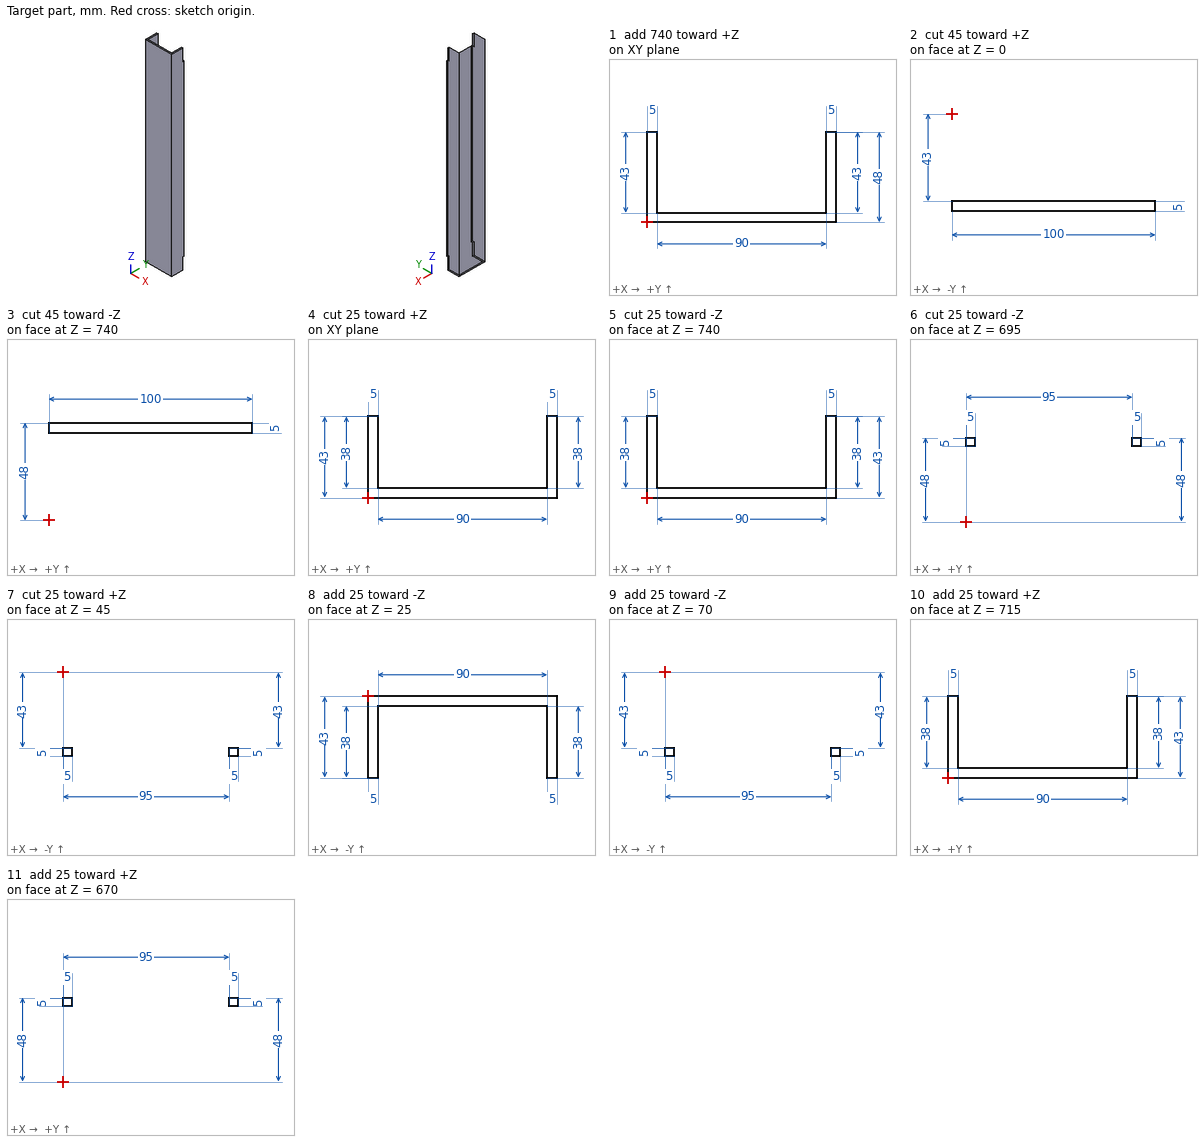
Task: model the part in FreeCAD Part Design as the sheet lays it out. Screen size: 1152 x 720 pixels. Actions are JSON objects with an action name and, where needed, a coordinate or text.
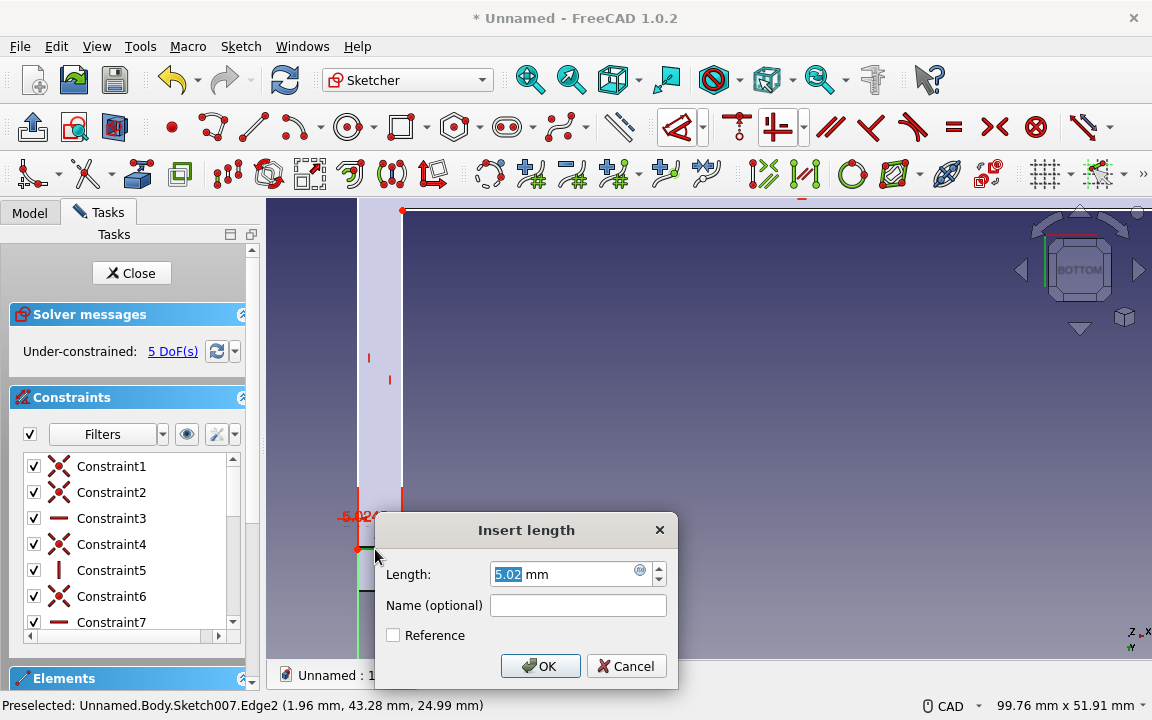
{"action": "type", "text": "5"}
{"action": "key", "text": "Return"}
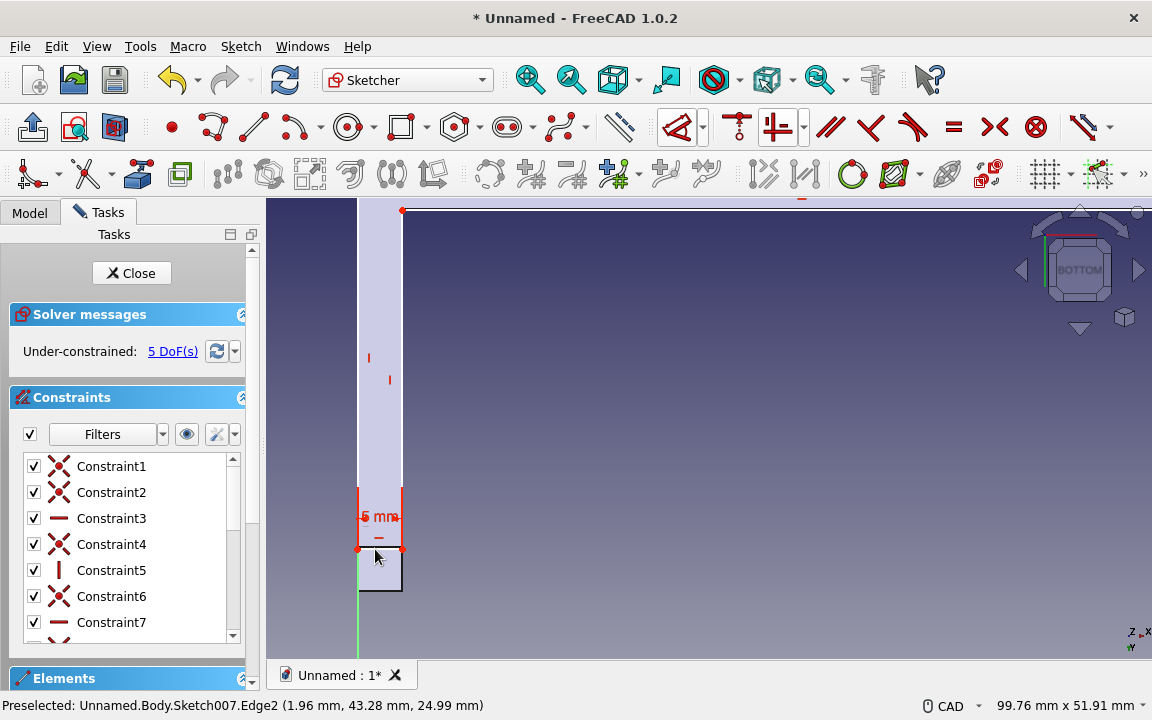
{"action": "scroll", "coordinate": [444, 517], "scroll_direction": "down", "scroll_amount": 3}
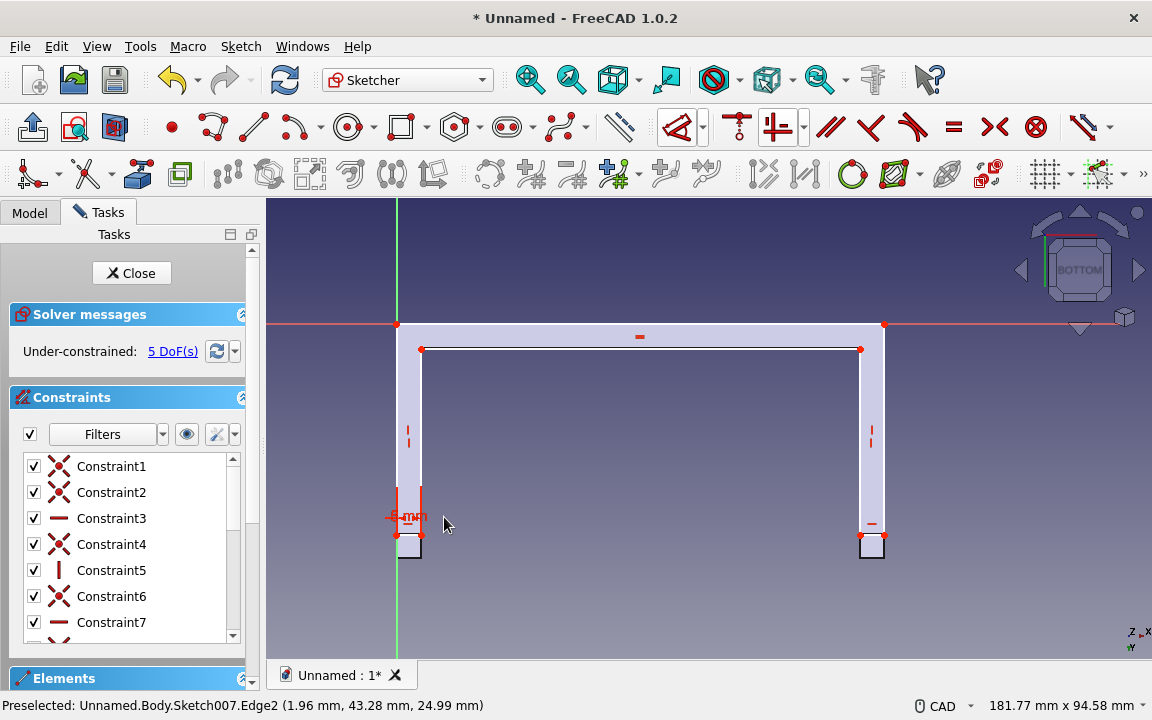
{"action": "scroll", "coordinate": [867, 535], "scroll_direction": "up", "scroll_amount": 4}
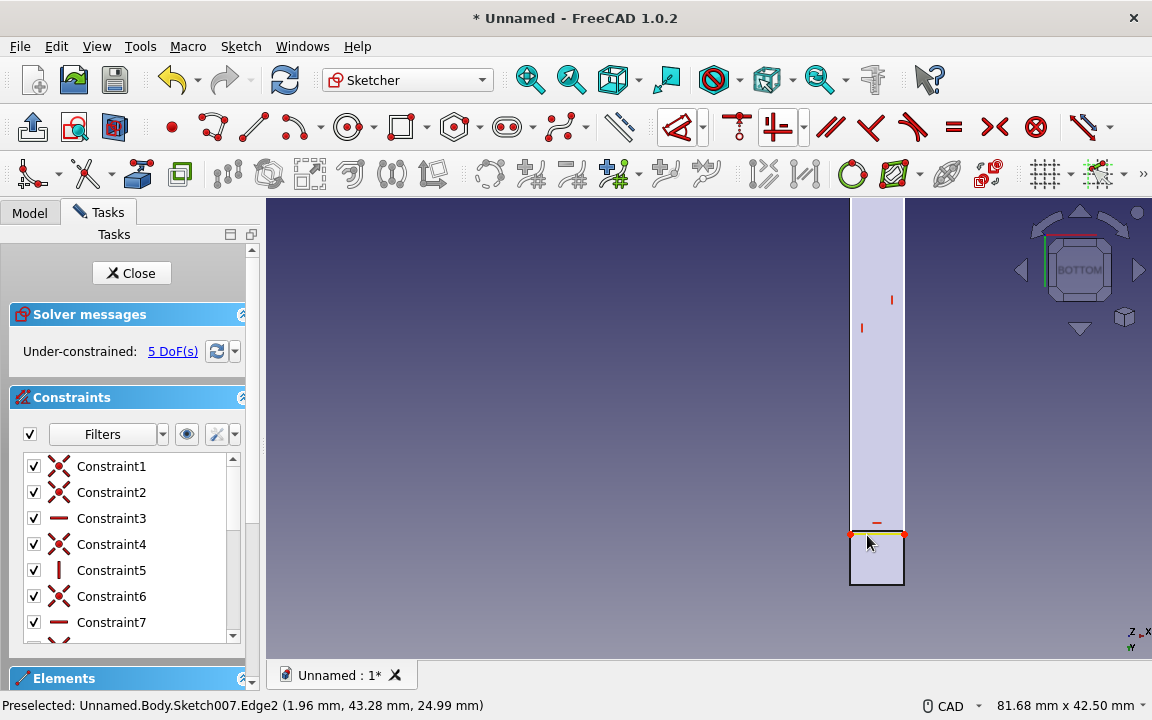
{"action": "left_click", "coordinate": [867, 534]}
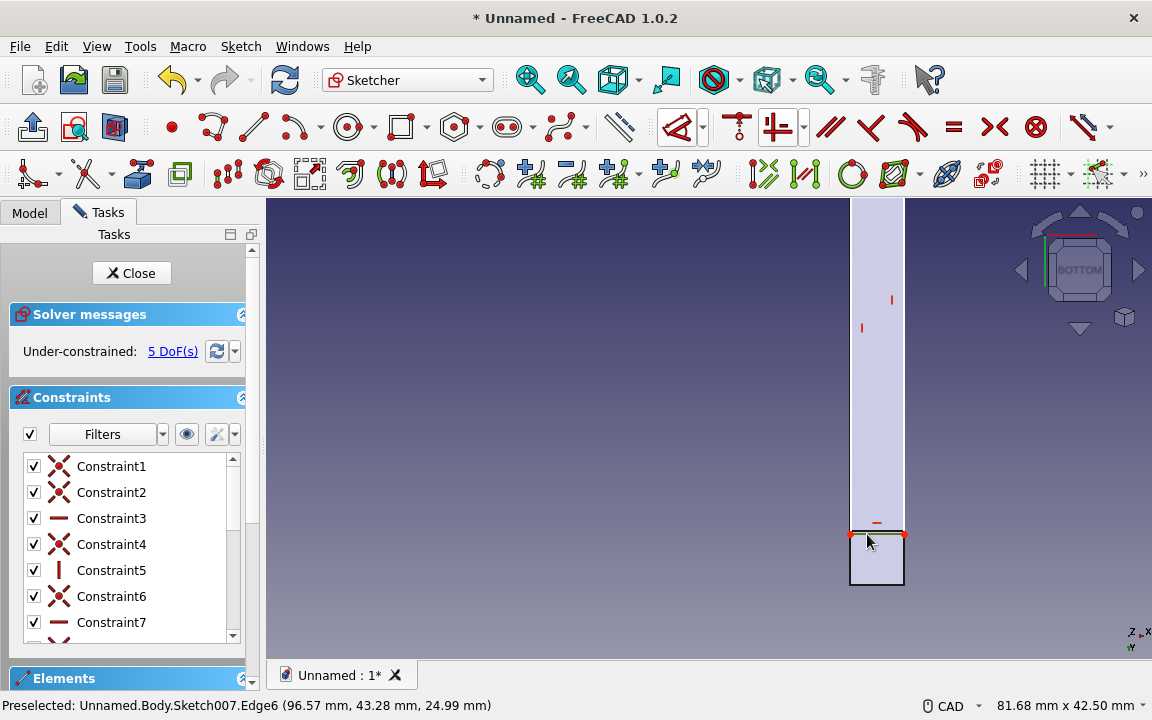
{"action": "left_click", "coordinate": [702, 128]}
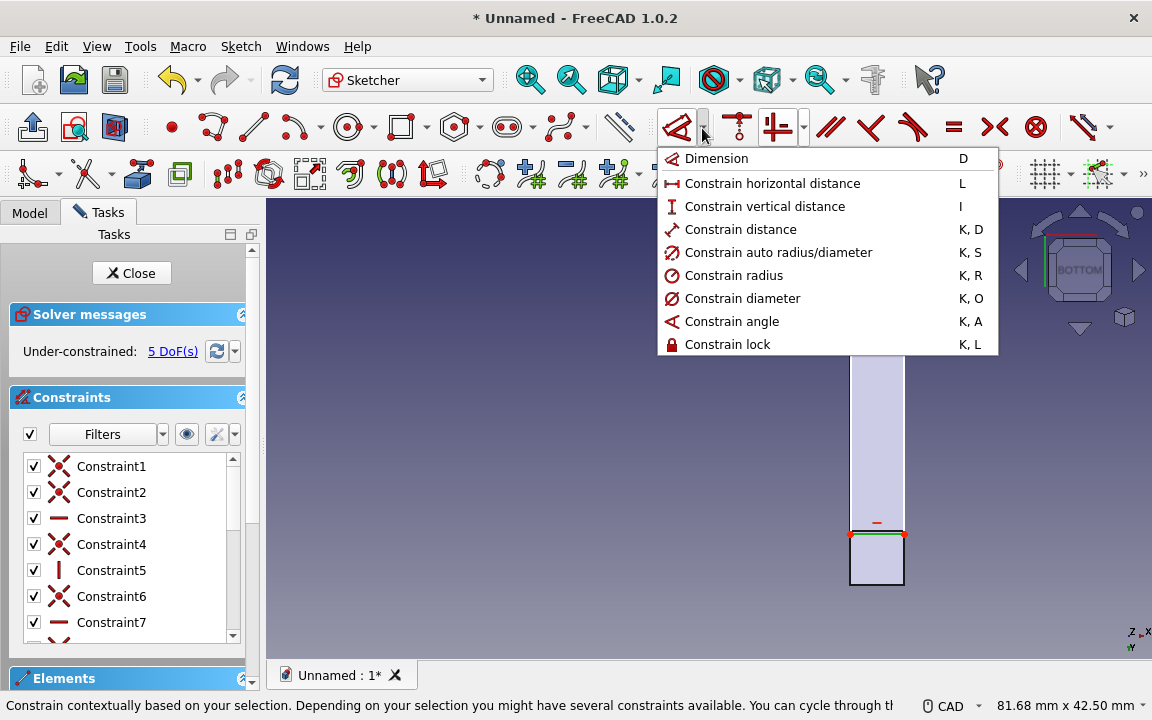
{"action": "left_click", "coordinate": [828, 184]}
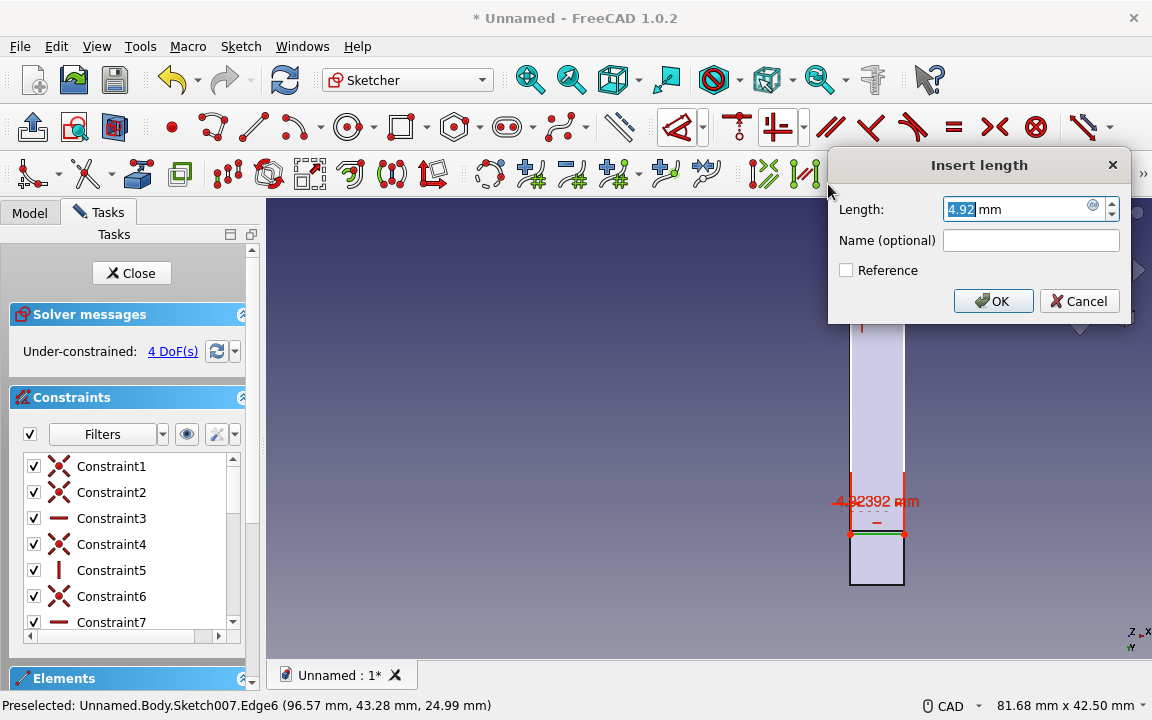
{"action": "type", "text": "5"}
{"action": "key", "text": "Return"}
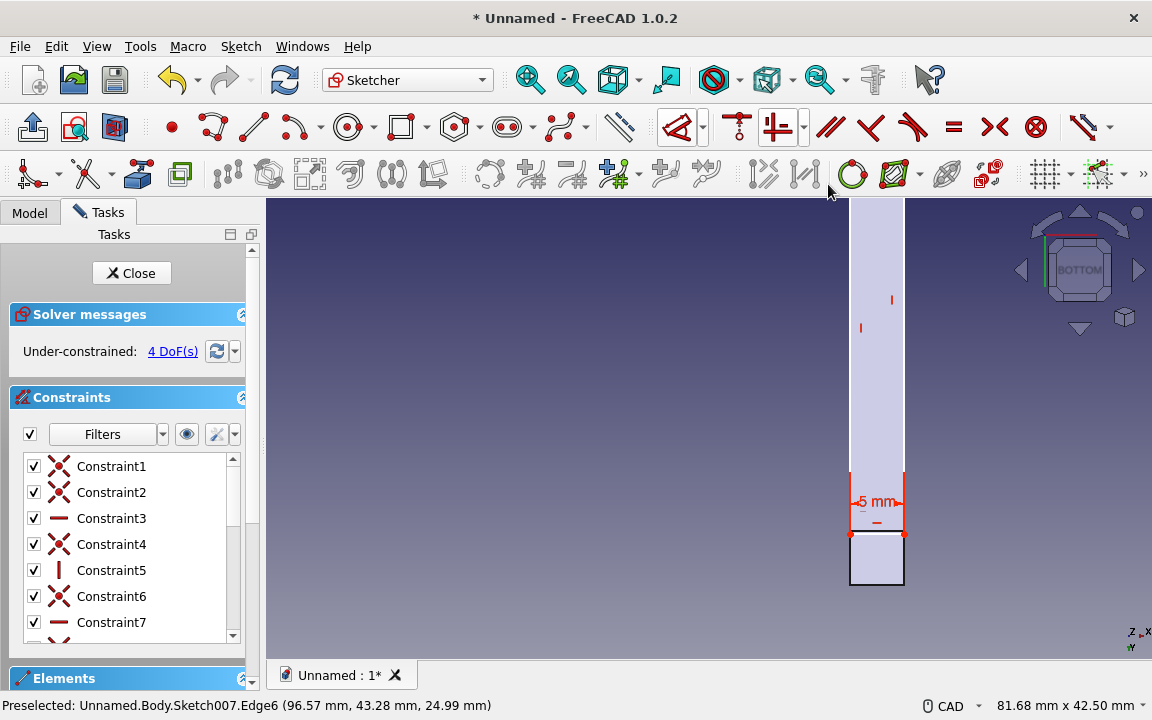
{"action": "scroll", "coordinate": [868, 535], "scroll_direction": "down", "scroll_amount": 4}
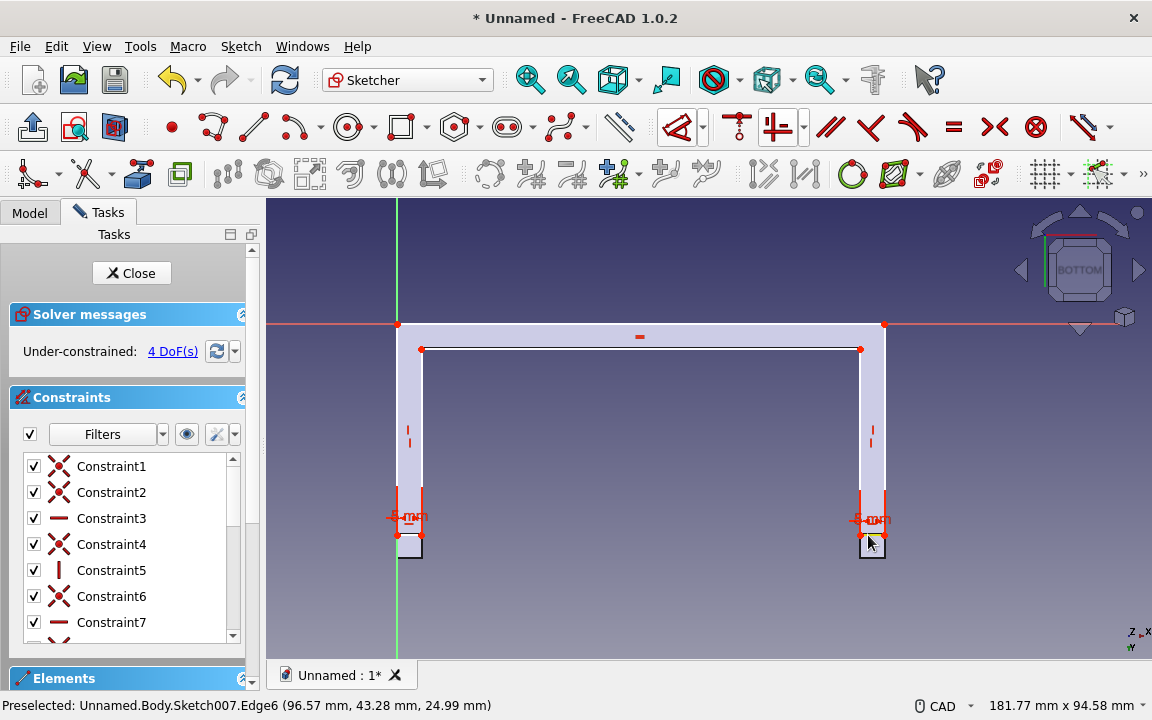
{"action": "left_click", "coordinate": [397, 387]}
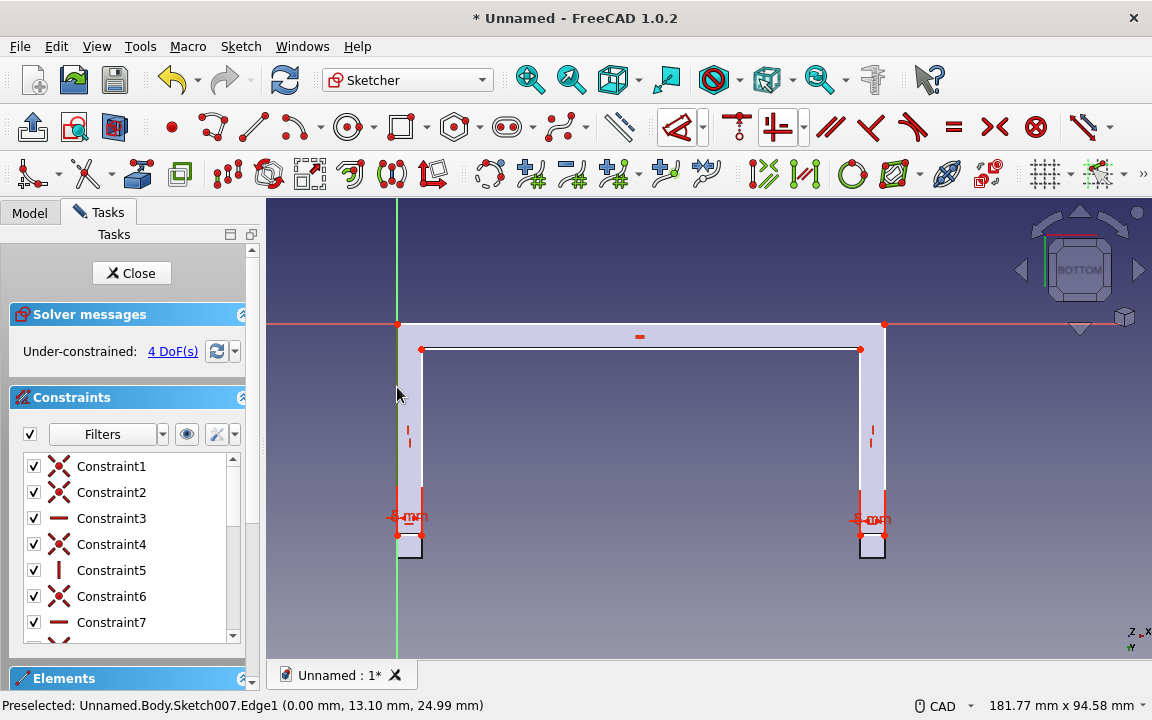
{"action": "left_click", "coordinate": [702, 128]}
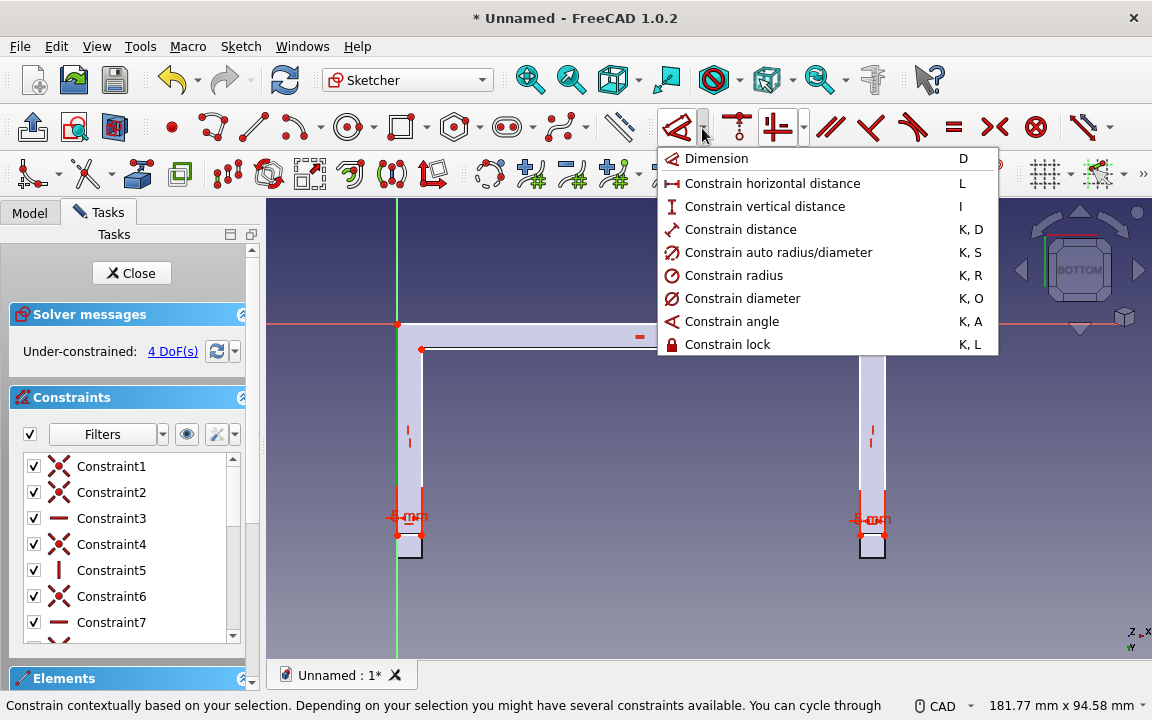
{"action": "left_click", "coordinate": [828, 206]}